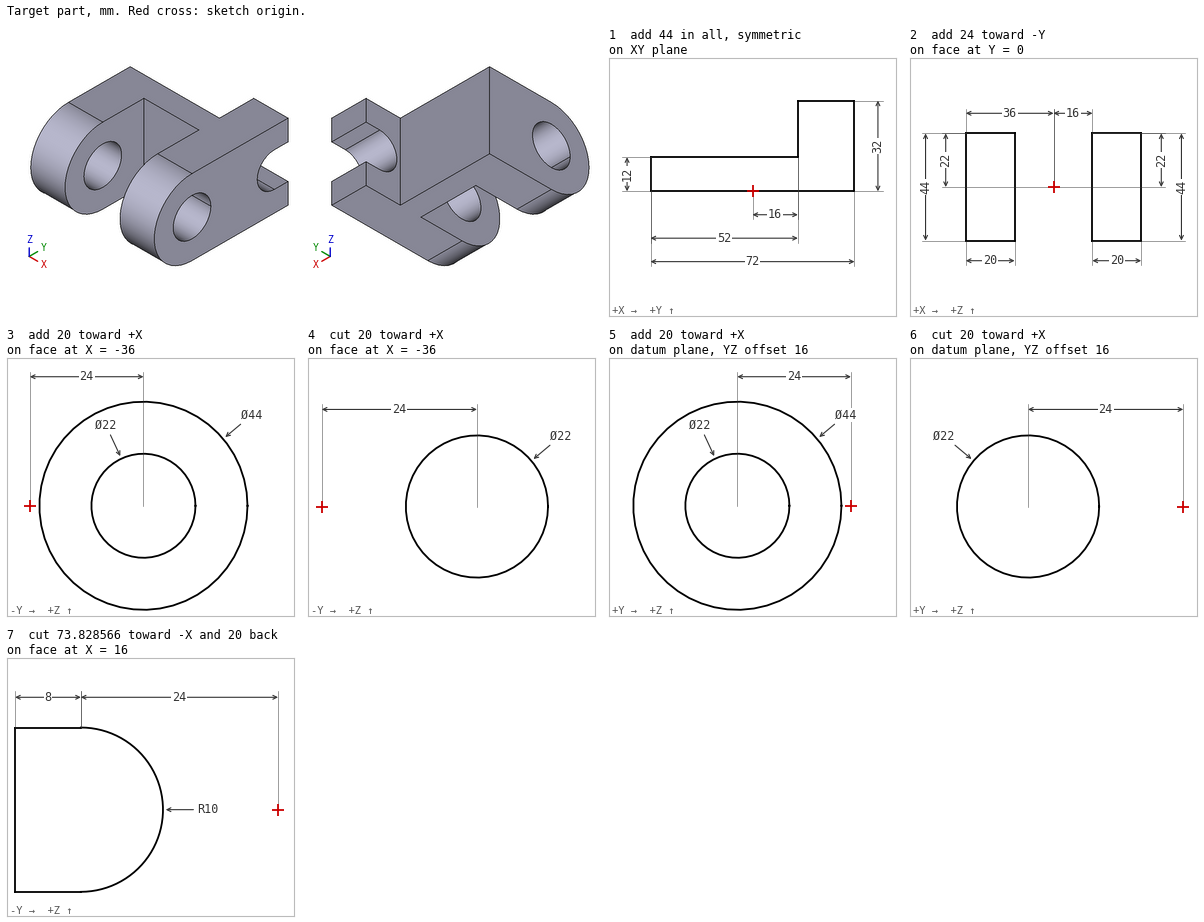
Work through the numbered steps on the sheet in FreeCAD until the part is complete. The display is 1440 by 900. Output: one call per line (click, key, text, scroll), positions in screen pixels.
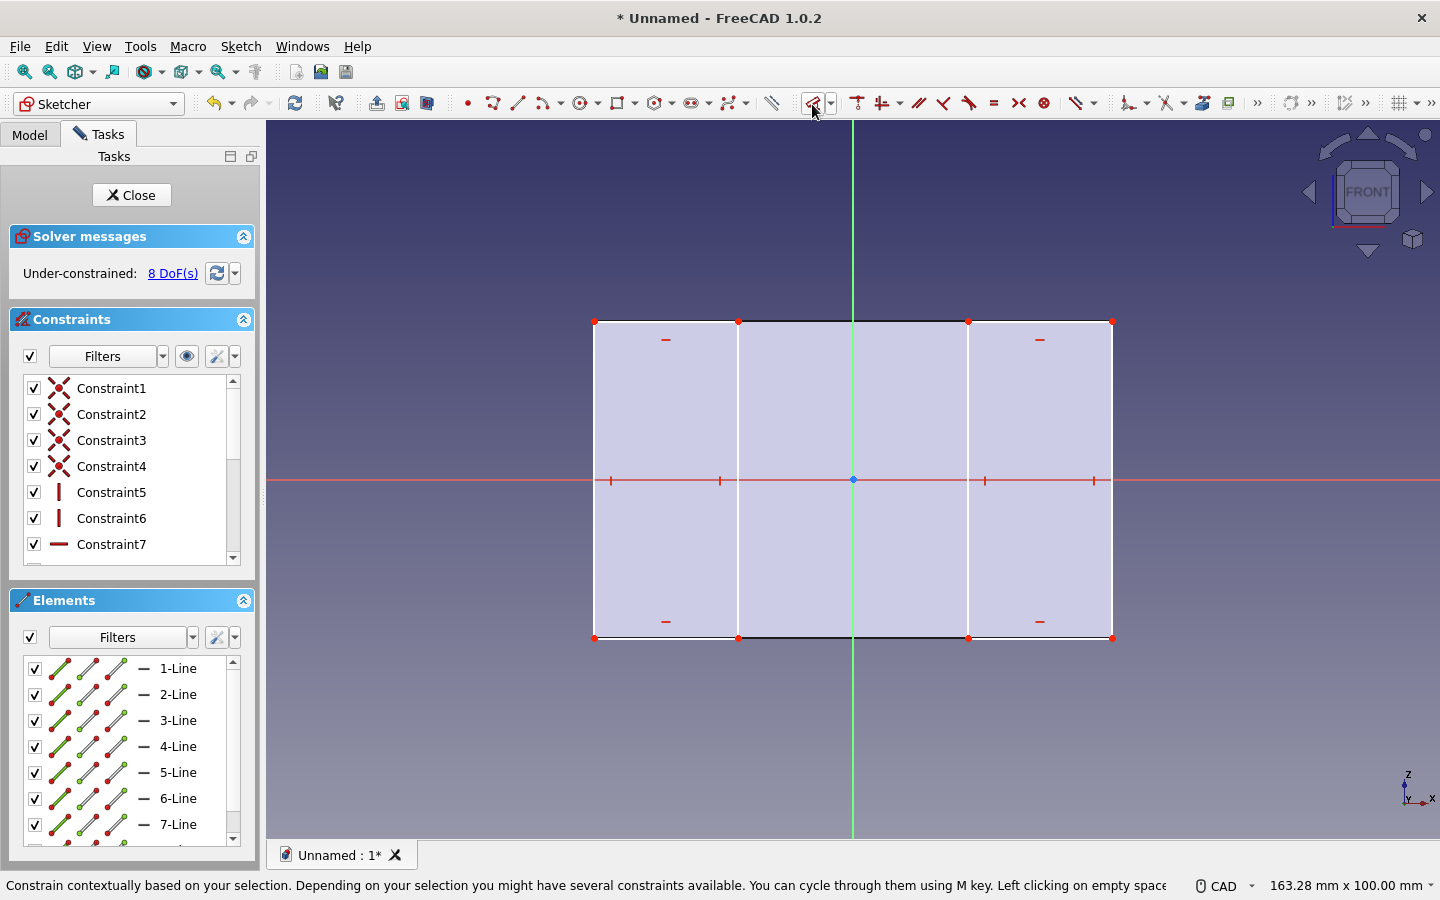
click(594, 417)
click(560, 408)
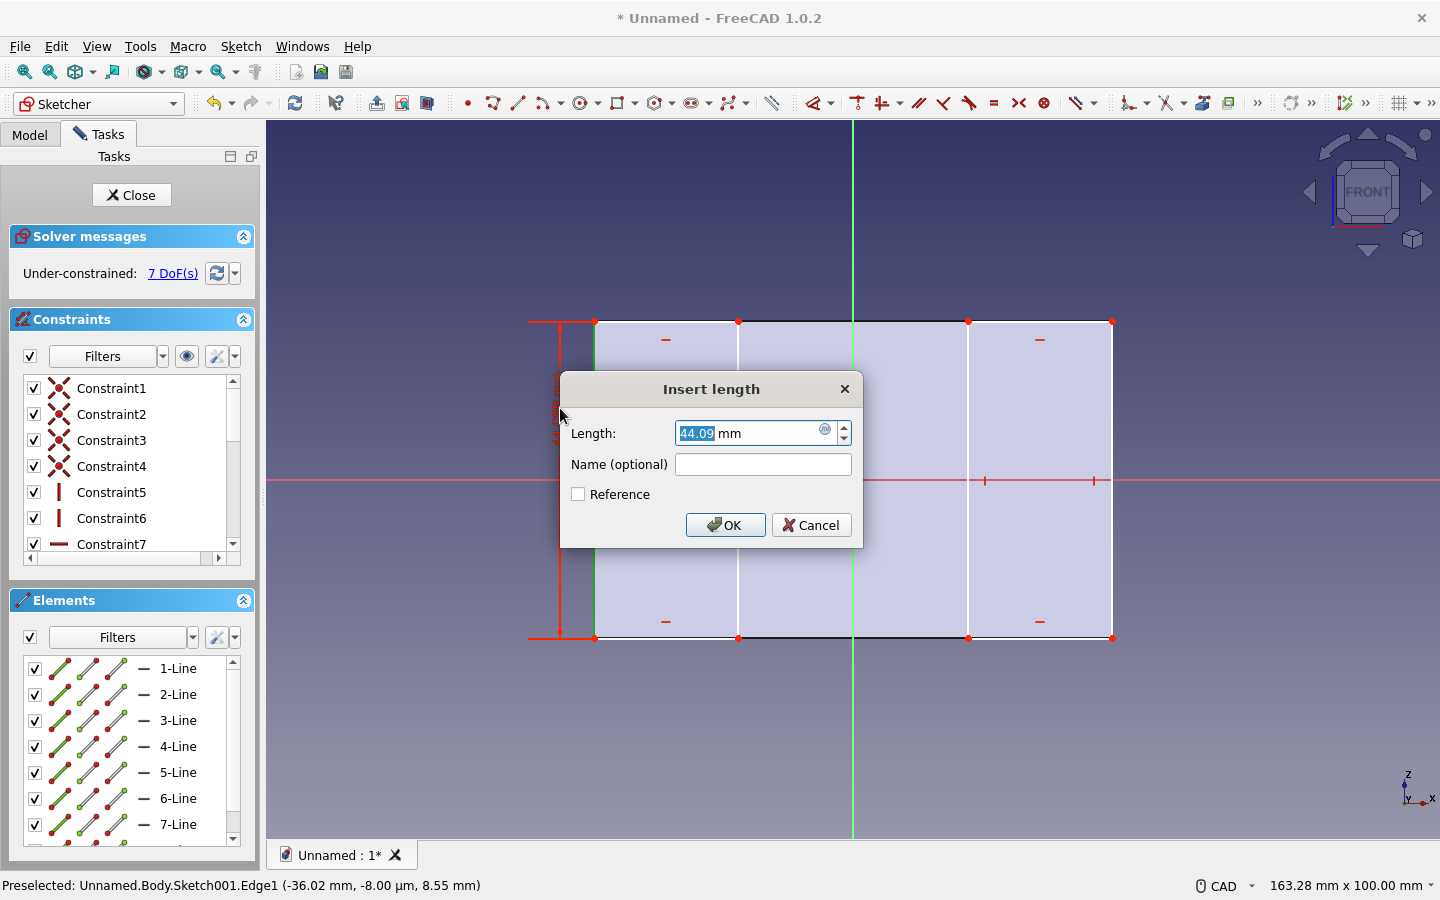
text(44)
key(Return)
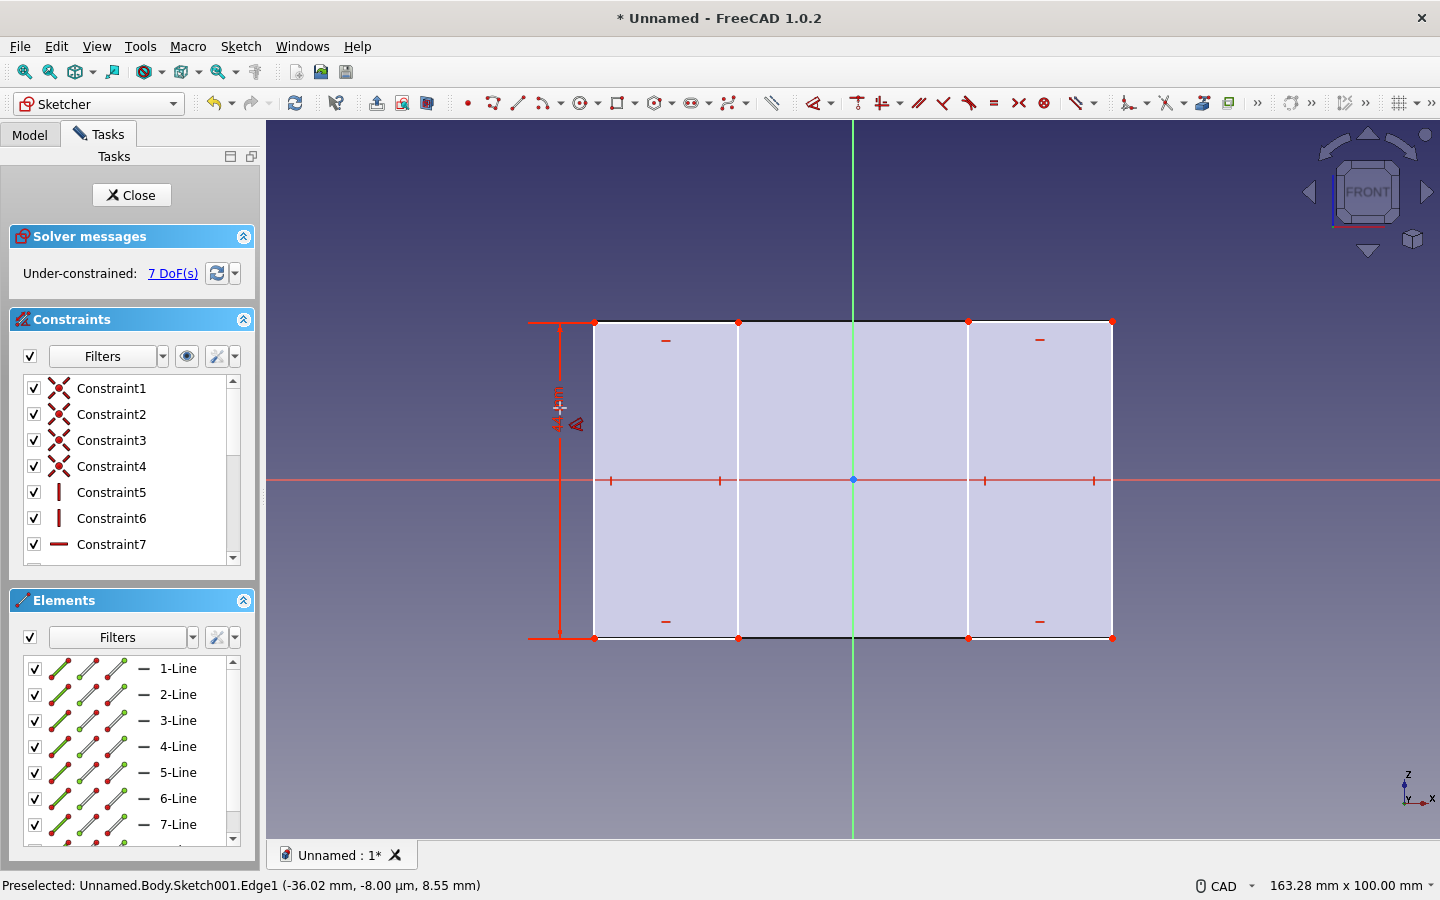
click(637, 639)
click(666, 673)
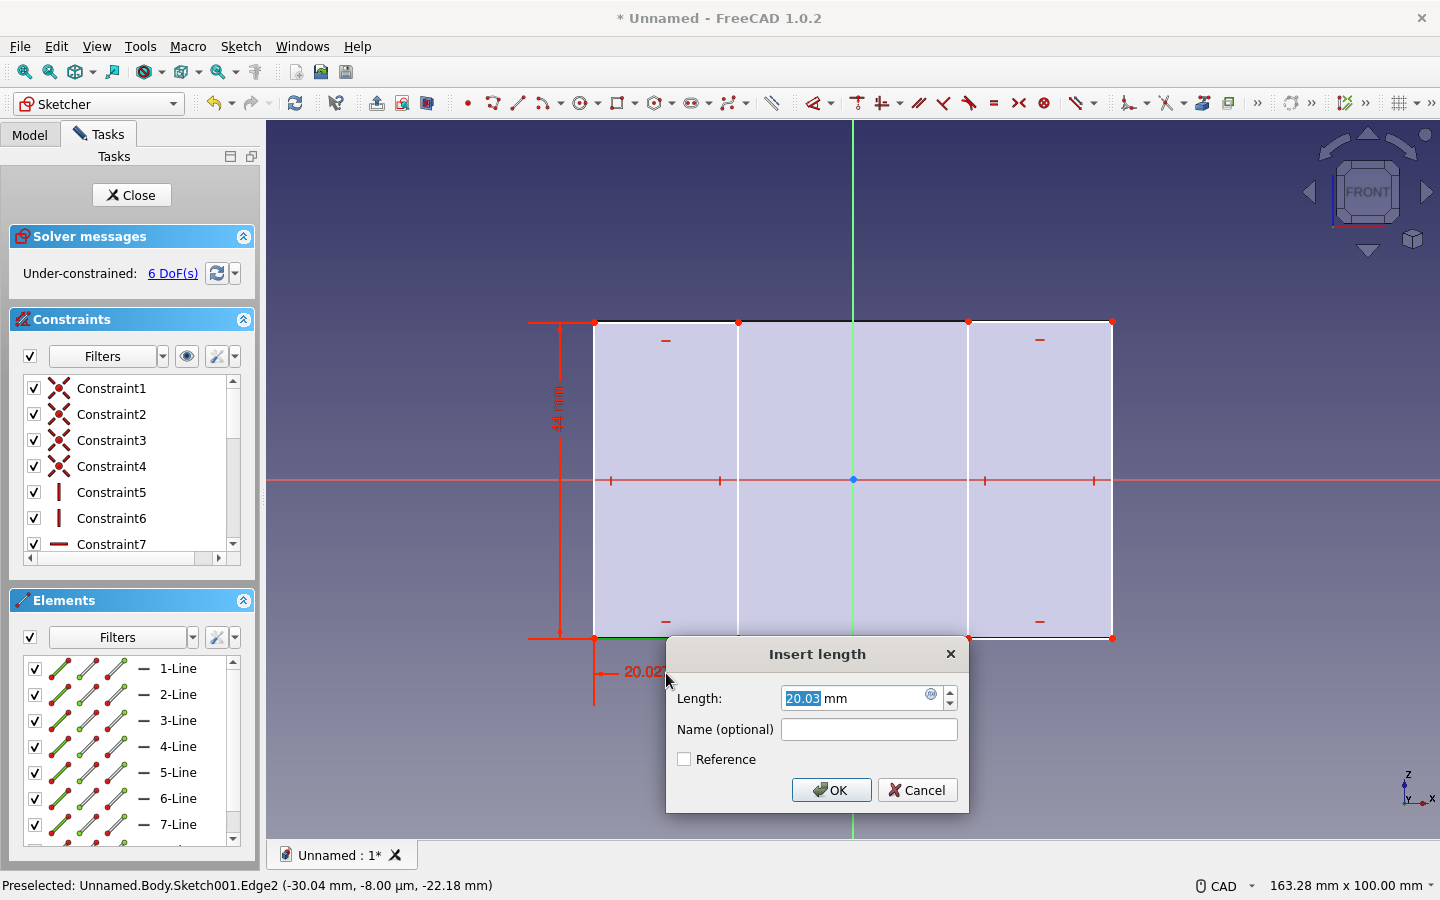
text(20)
key(Return)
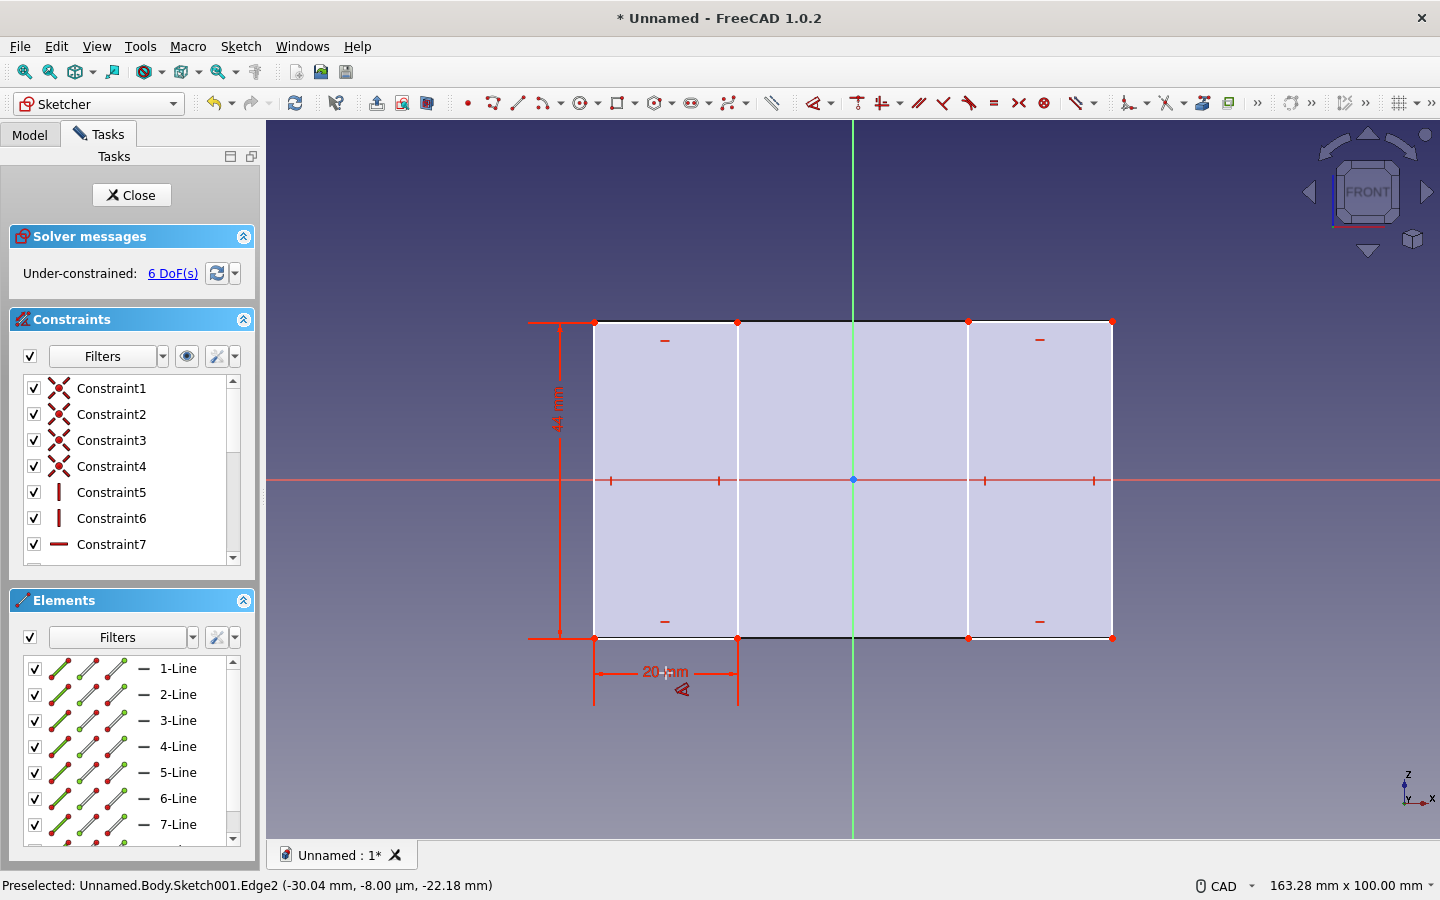
click(968, 417)
click(1002, 408)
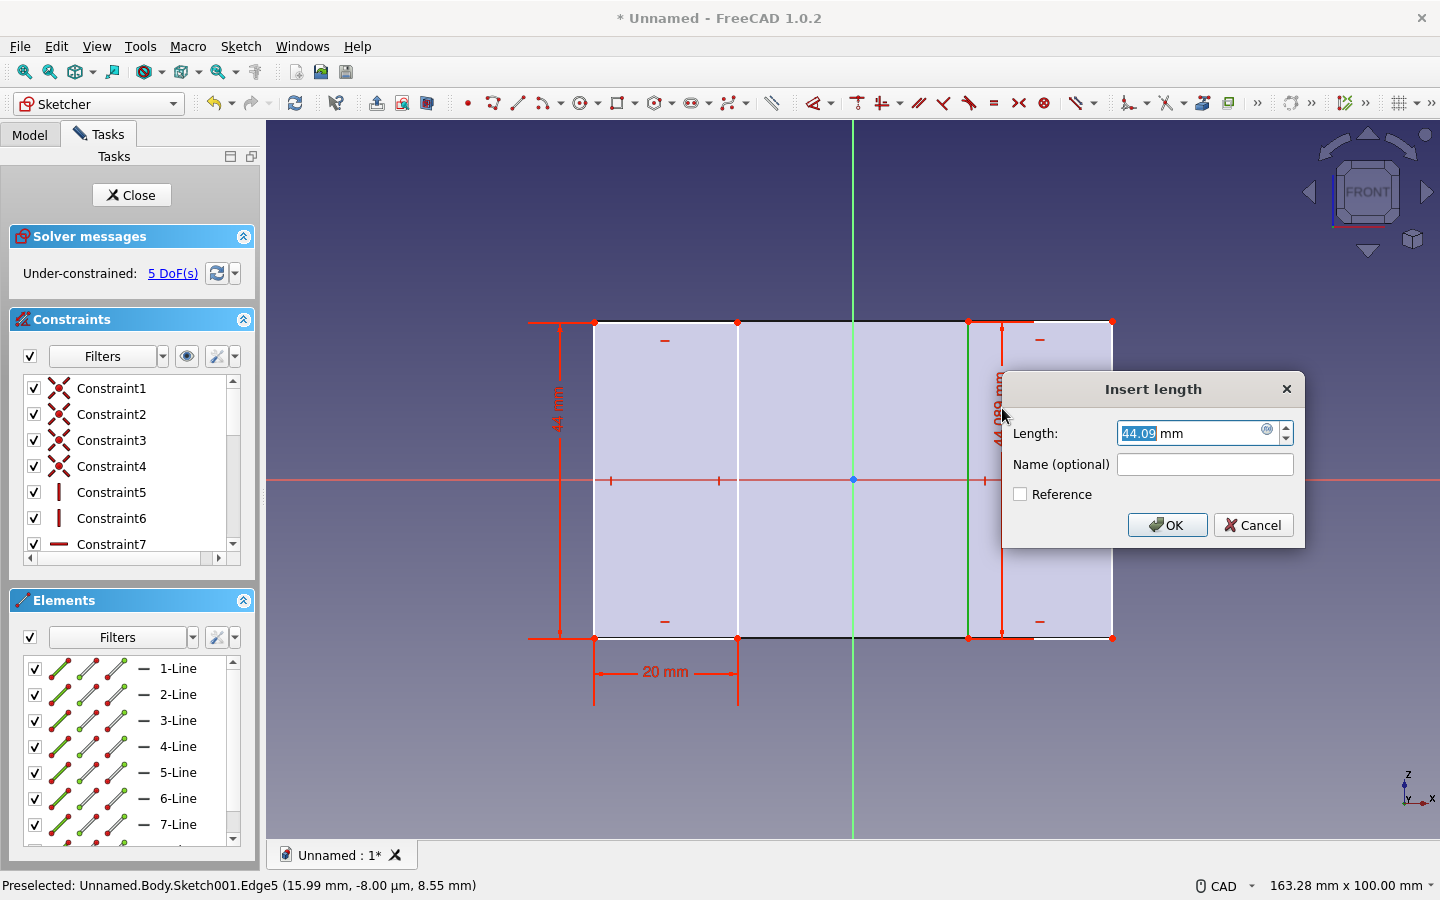
text(44)
key(Return)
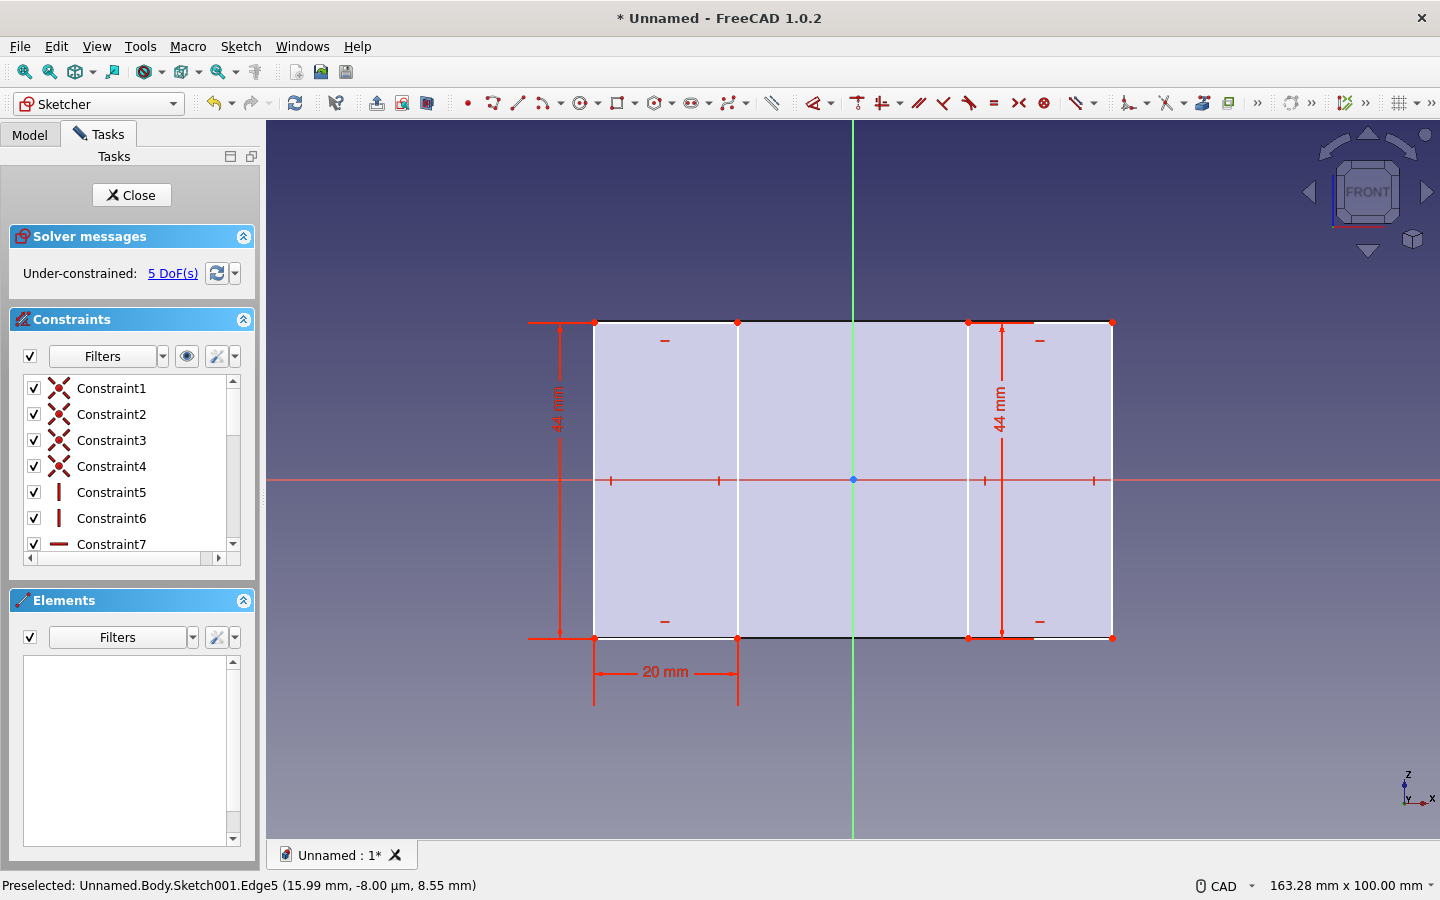
click(1011, 639)
click(1040, 673)